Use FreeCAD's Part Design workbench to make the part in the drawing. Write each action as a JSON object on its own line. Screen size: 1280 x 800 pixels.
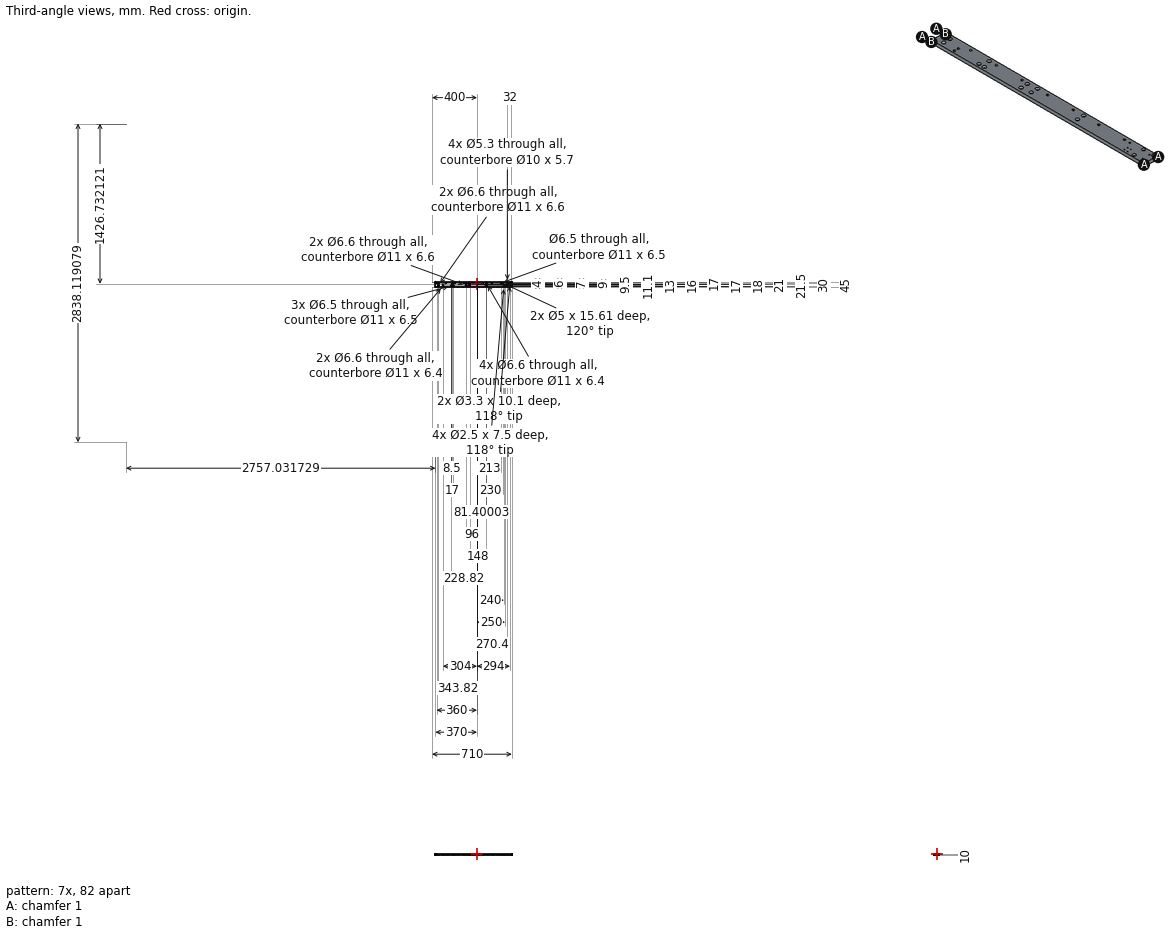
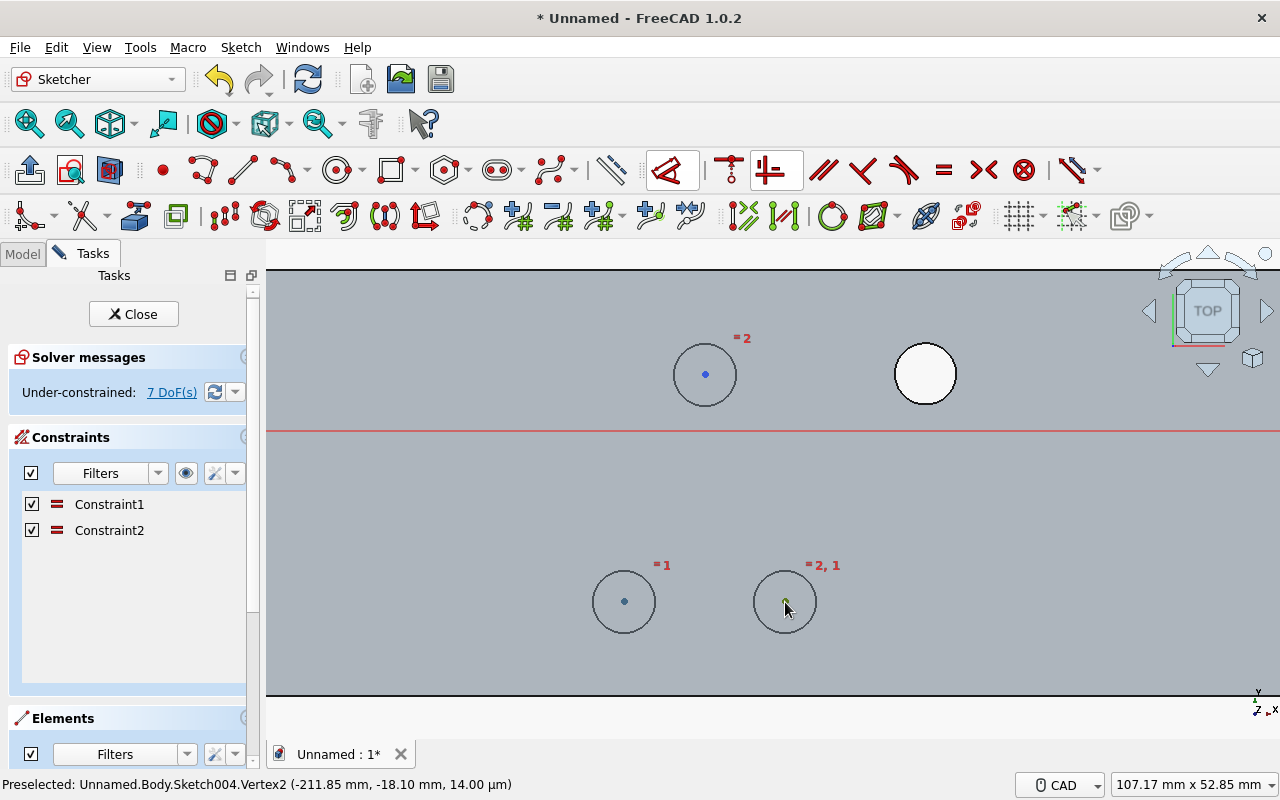
{"action": "left_click", "coordinate": [798, 170]}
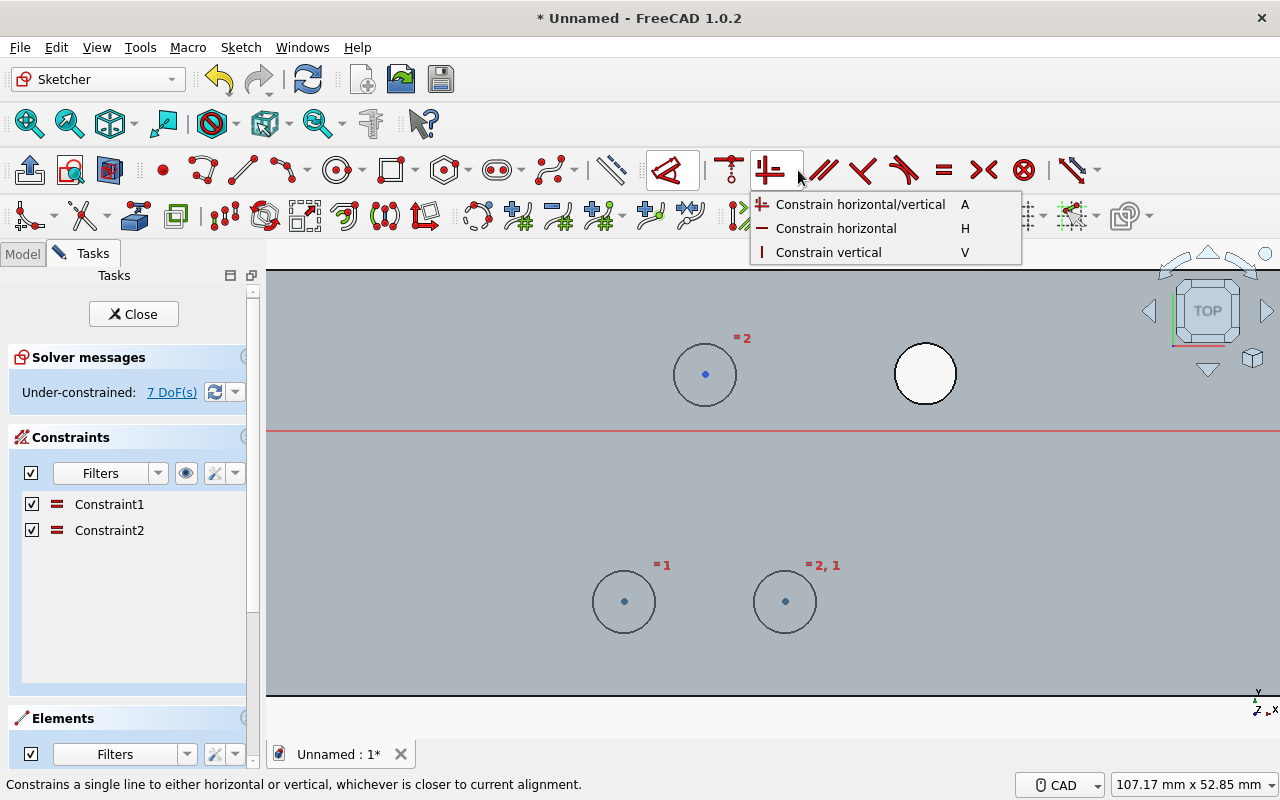
{"action": "left_click", "coordinate": [886, 228]}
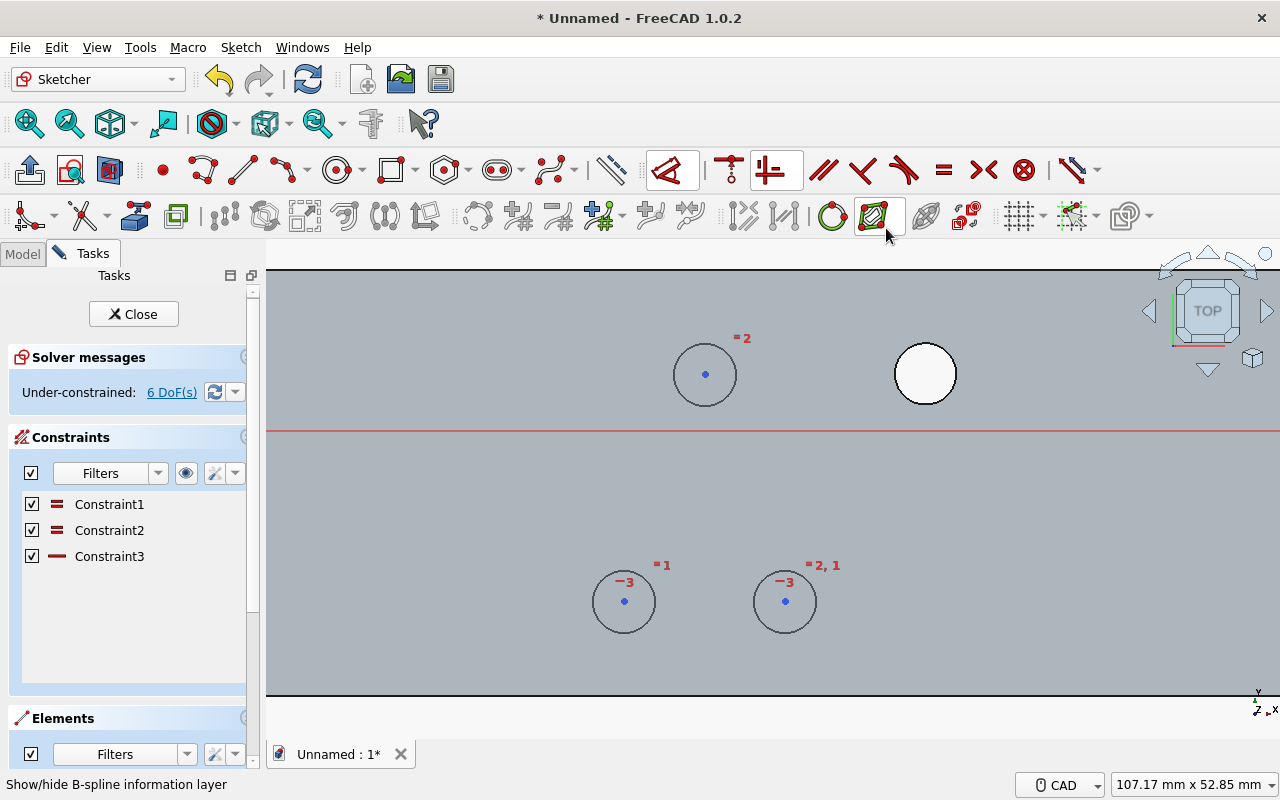
{"action": "left_click", "coordinate": [646, 580]}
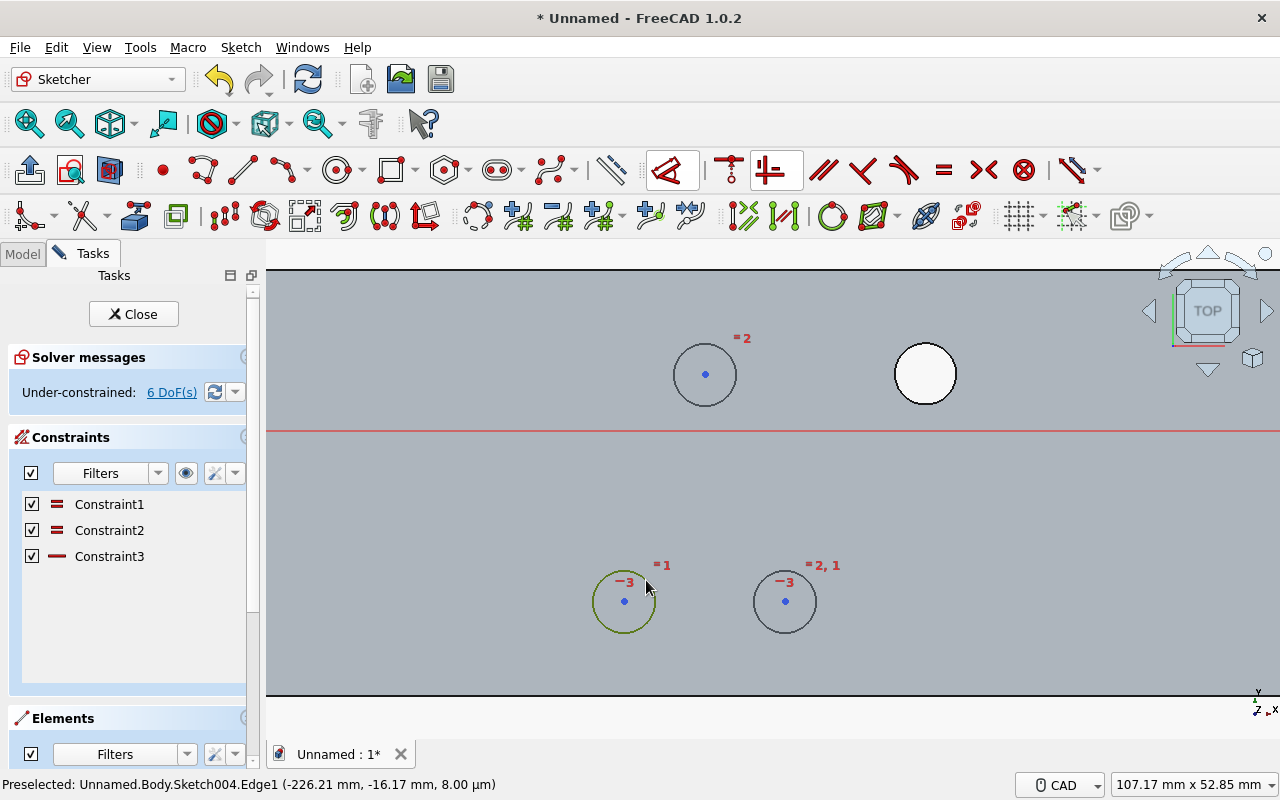
{"action": "left_click", "coordinate": [694, 170]}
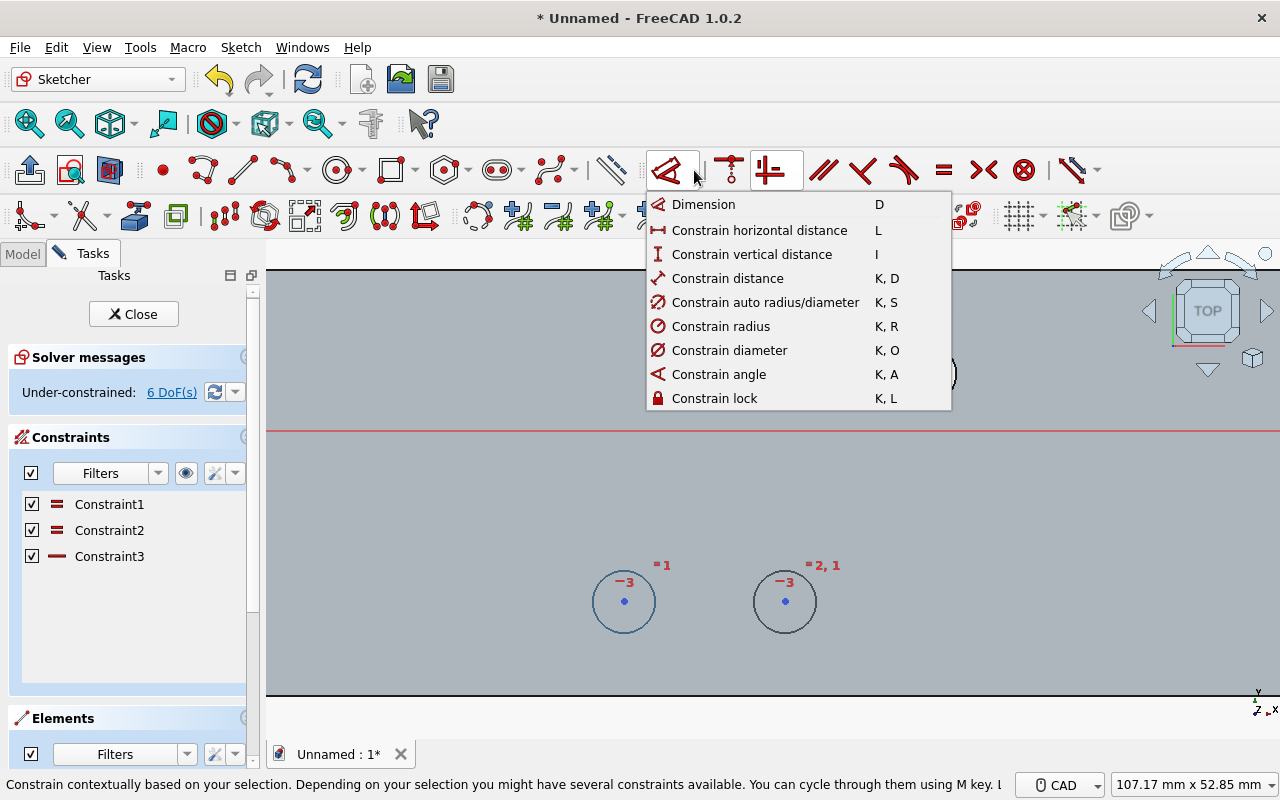
{"action": "left_click", "coordinate": [799, 350]}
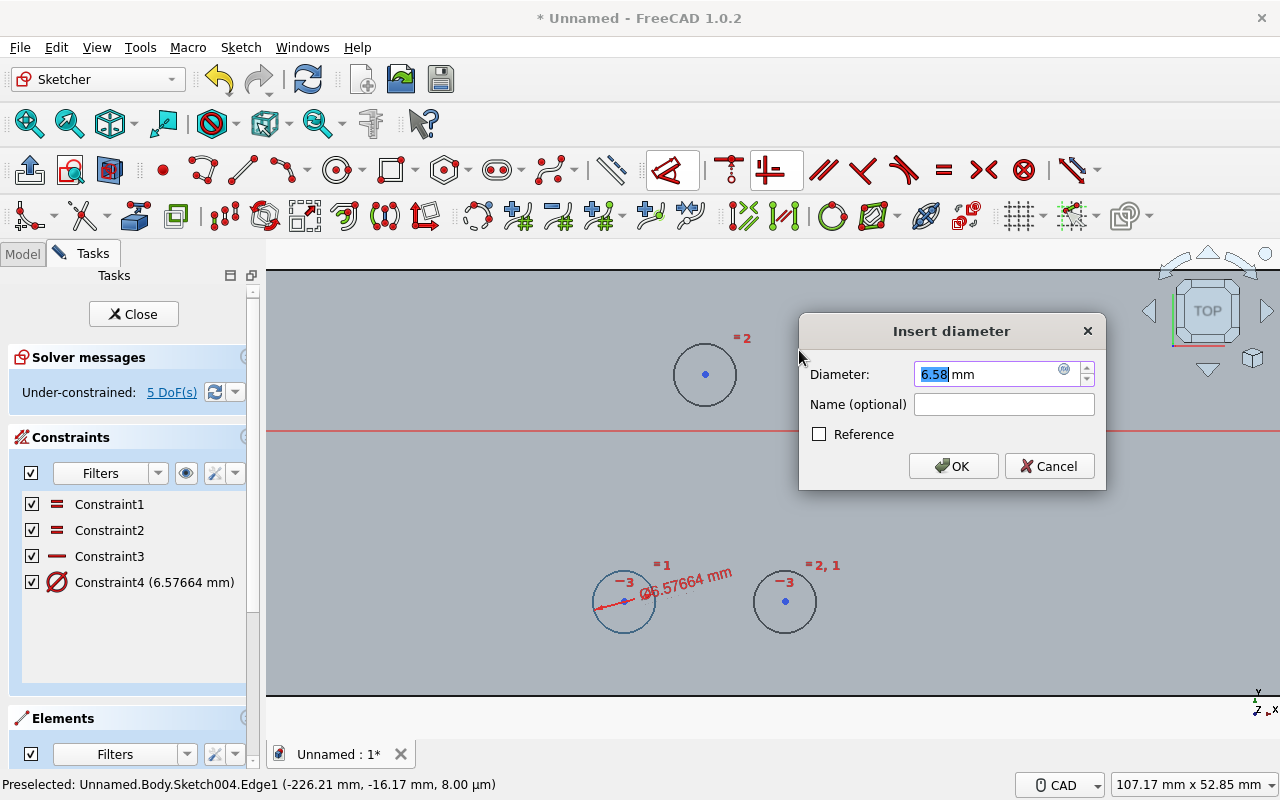
{"action": "type", "text": "6.5"}
{"action": "key", "text": "Return"}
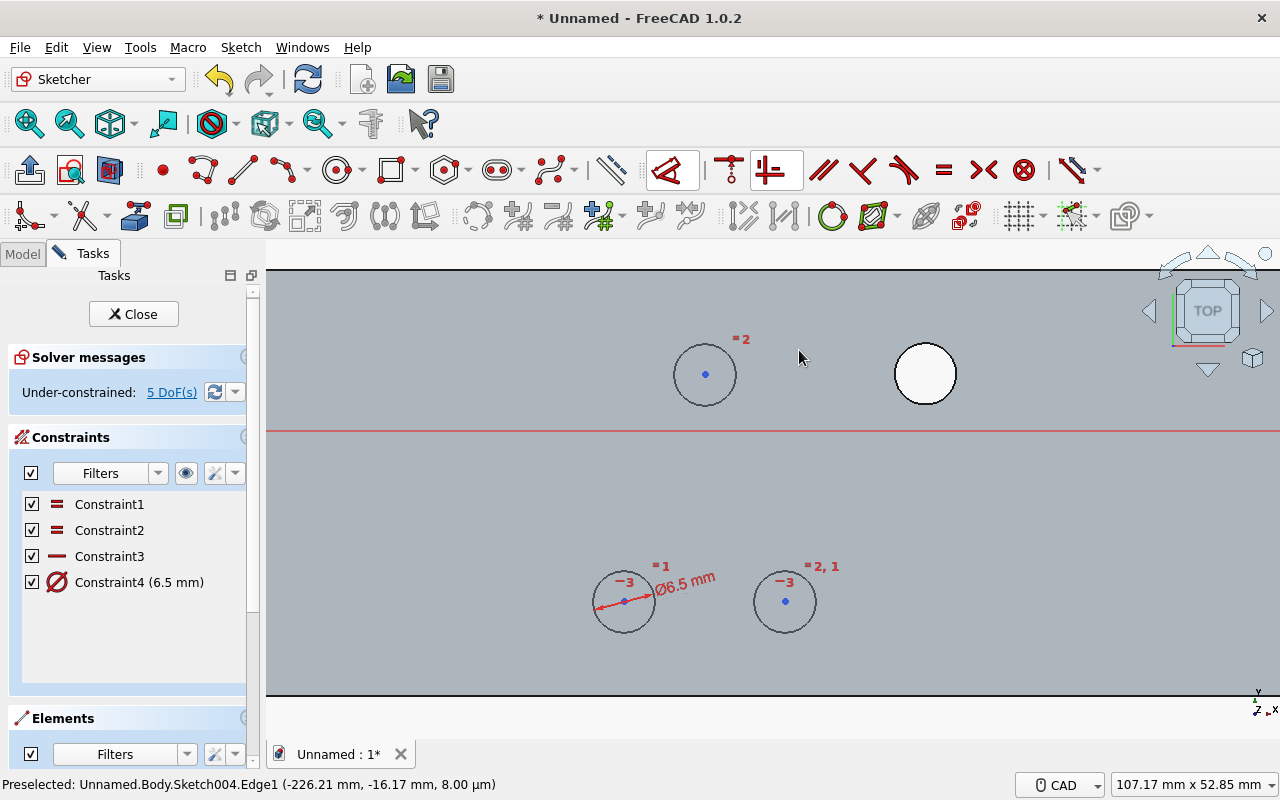
{"action": "left_click", "coordinate": [705, 375]}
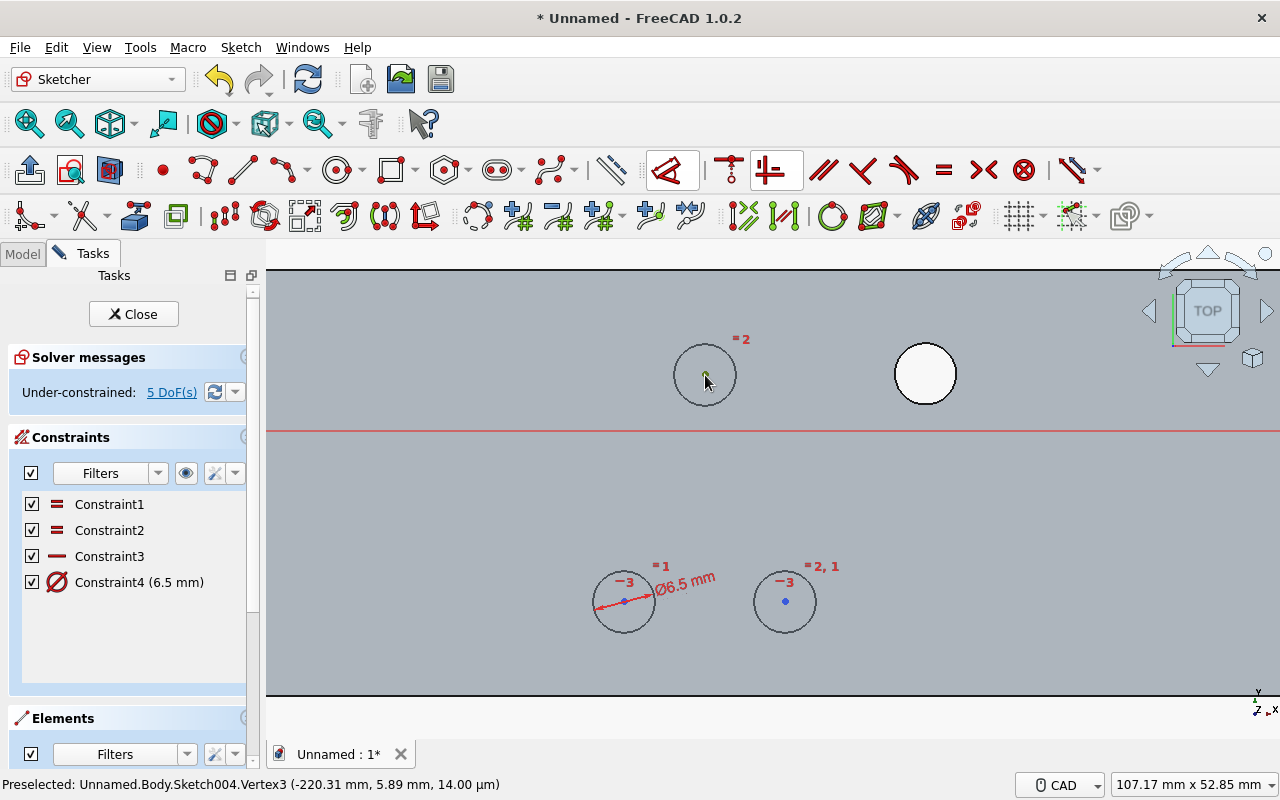
{"action": "key", "text": "i"}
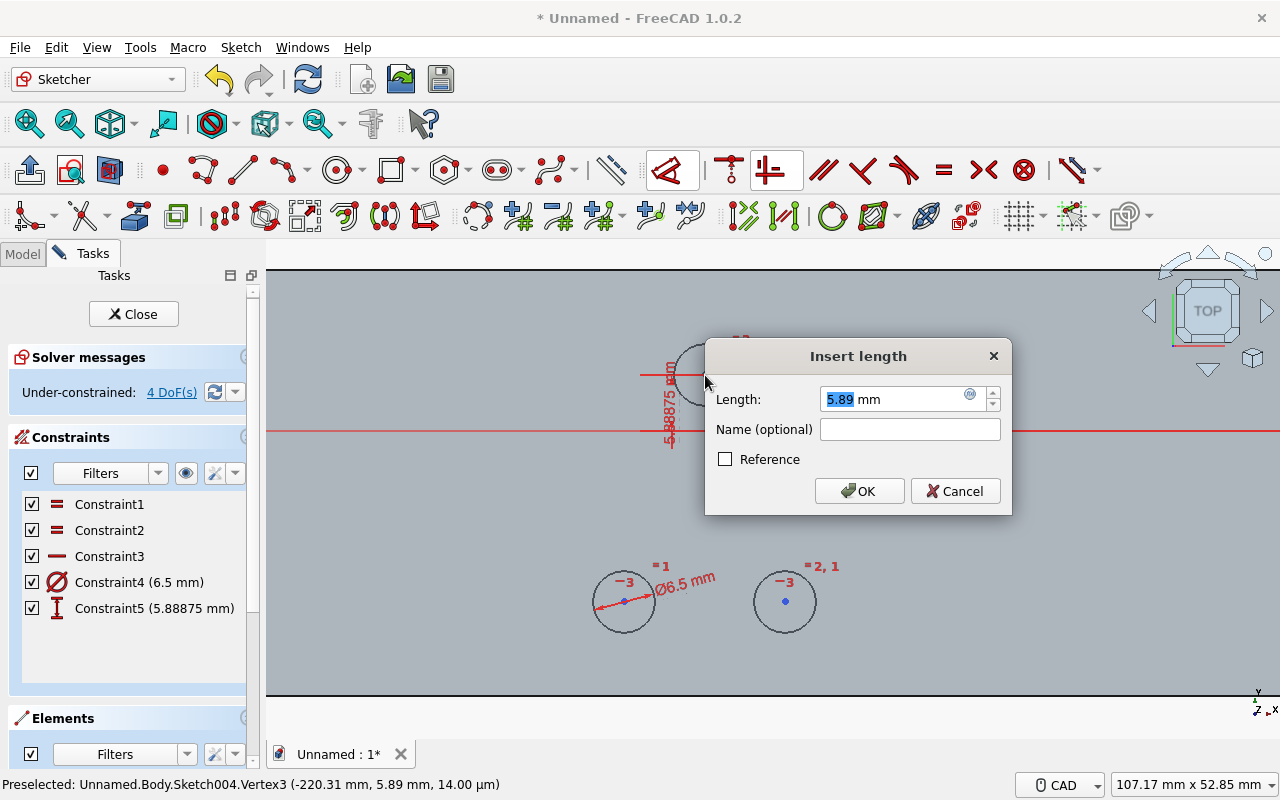
{"action": "type", "text": "6"}
{"action": "key", "text": "Return"}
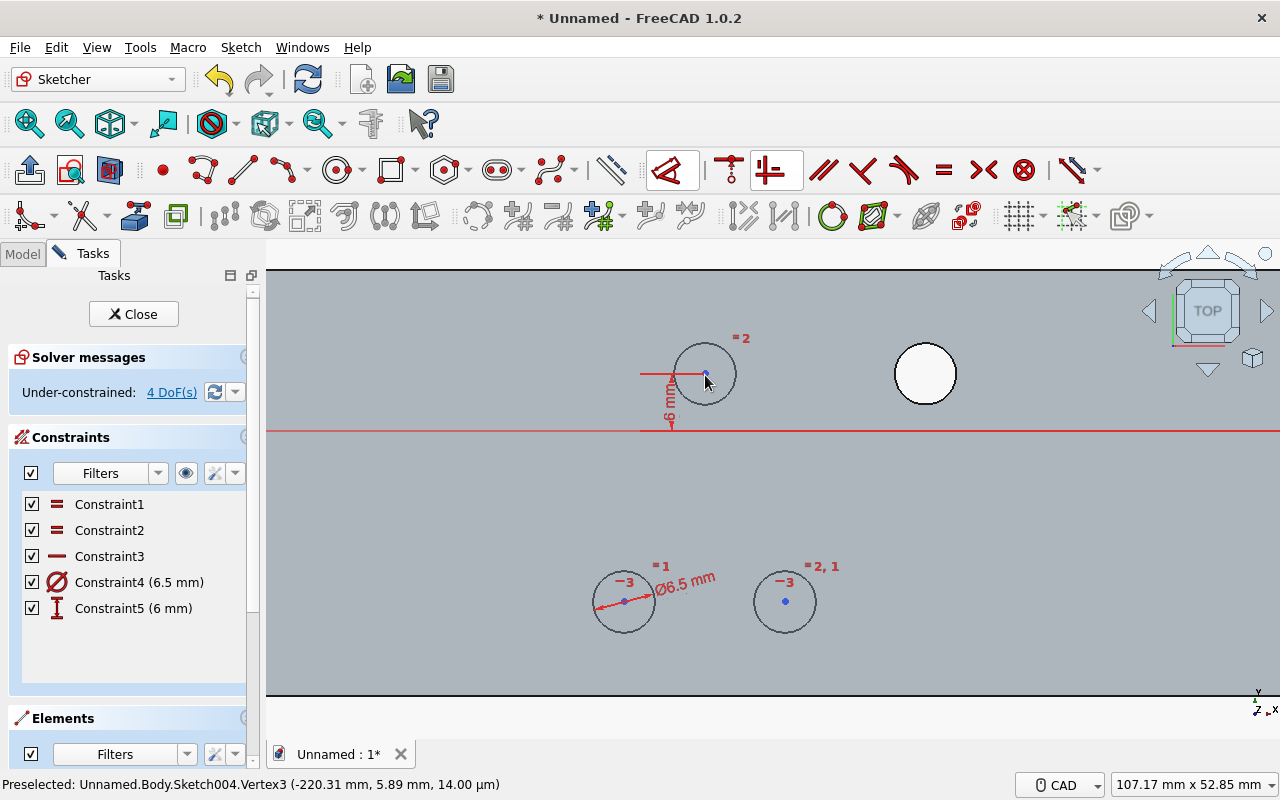
{"action": "left_click", "coordinate": [624, 602]}